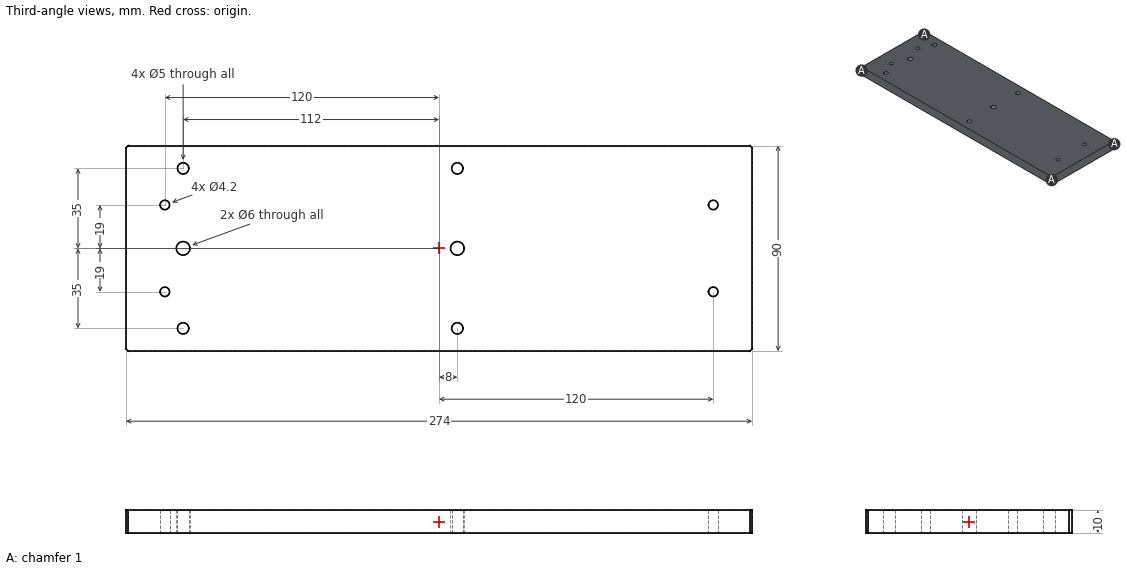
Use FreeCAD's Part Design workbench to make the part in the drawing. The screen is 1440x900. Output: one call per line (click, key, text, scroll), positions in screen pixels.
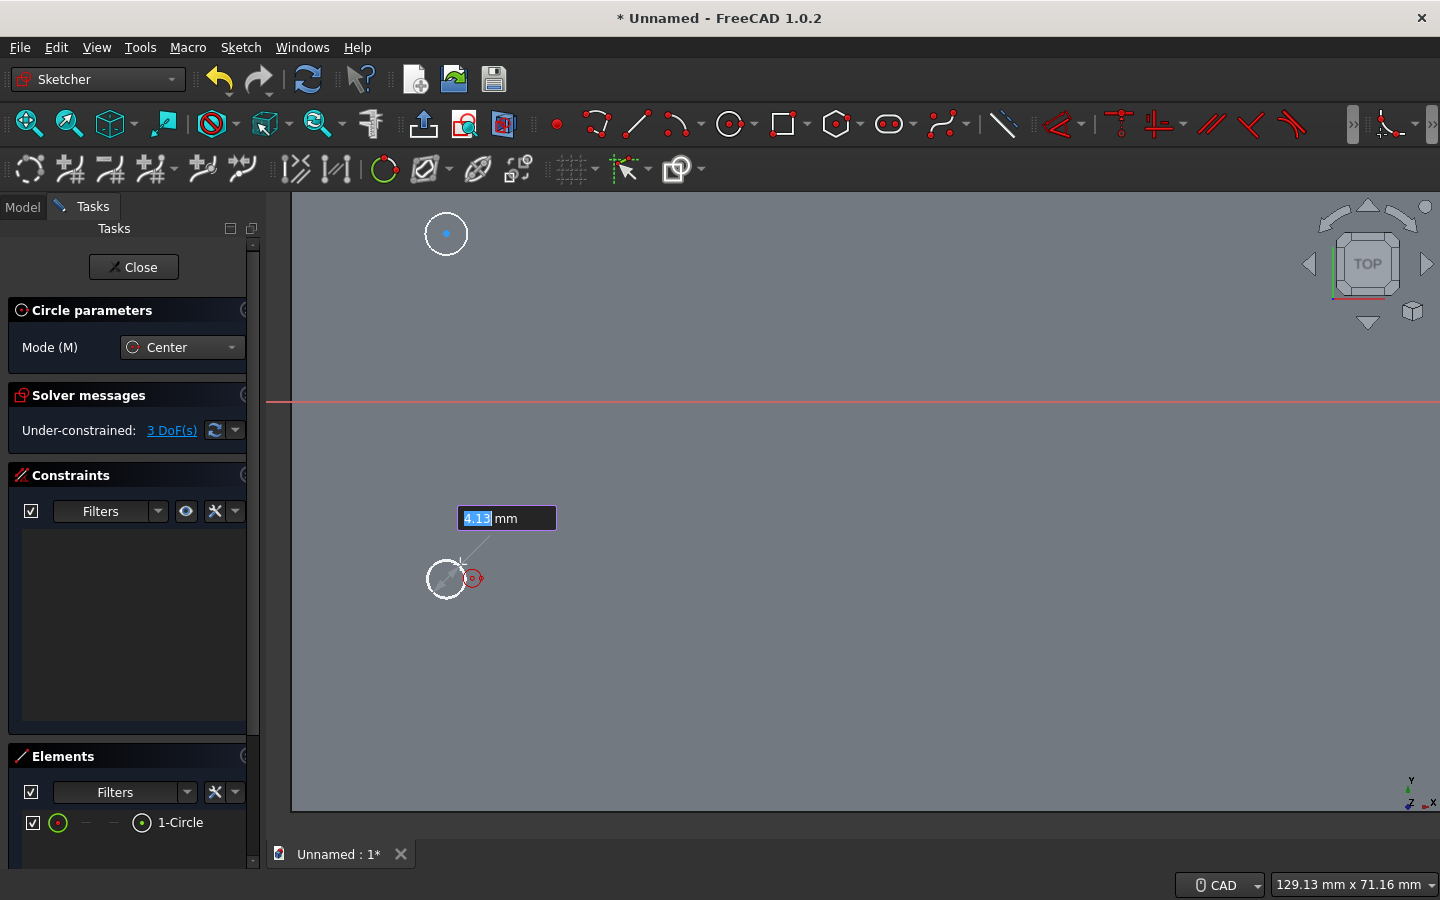
click(459, 562)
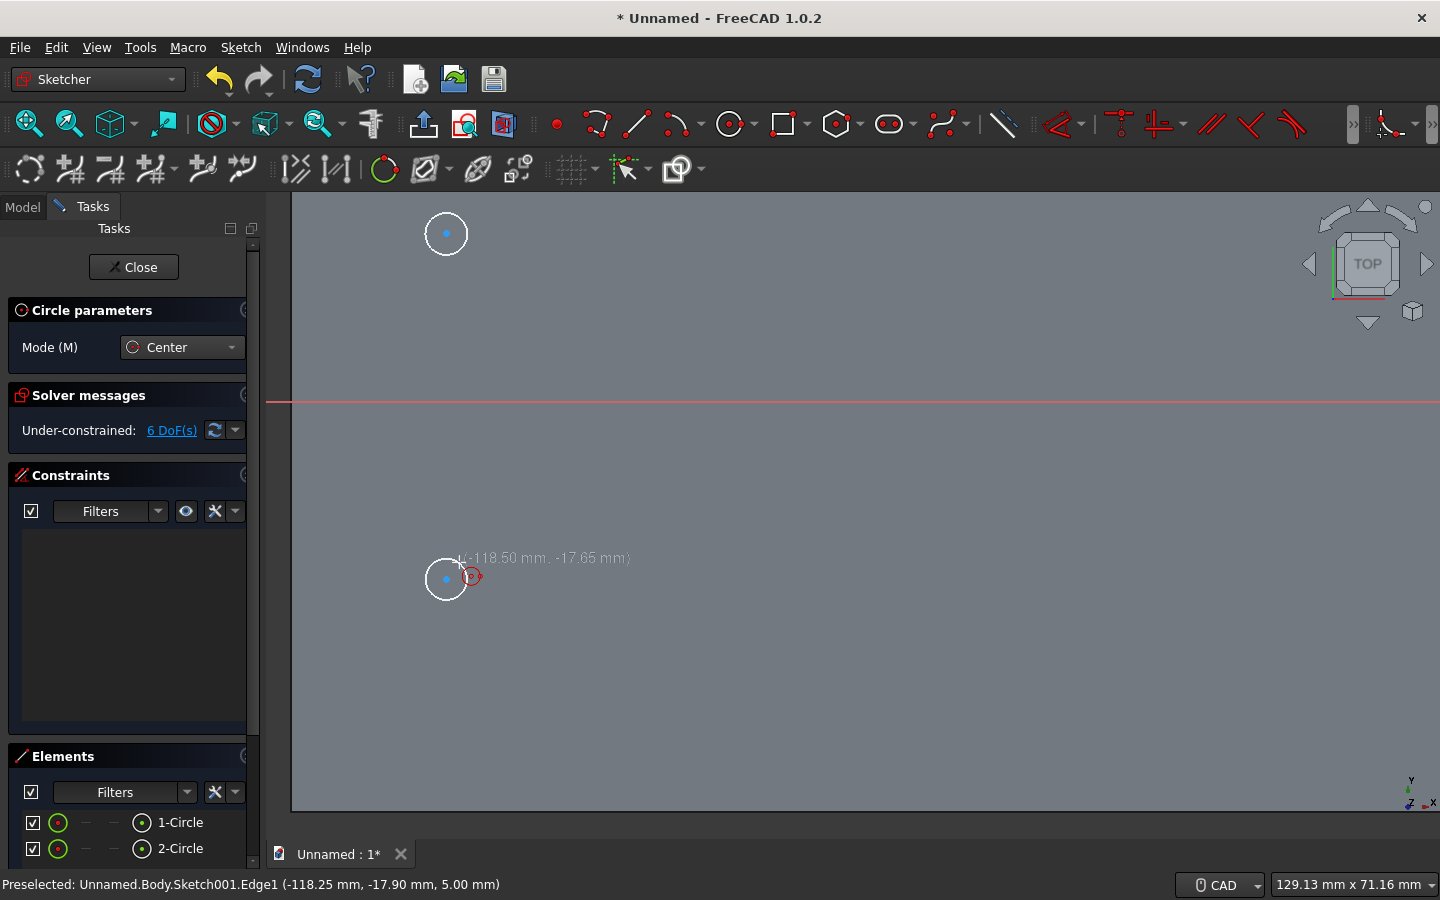
scroll(460, 564, down, 6)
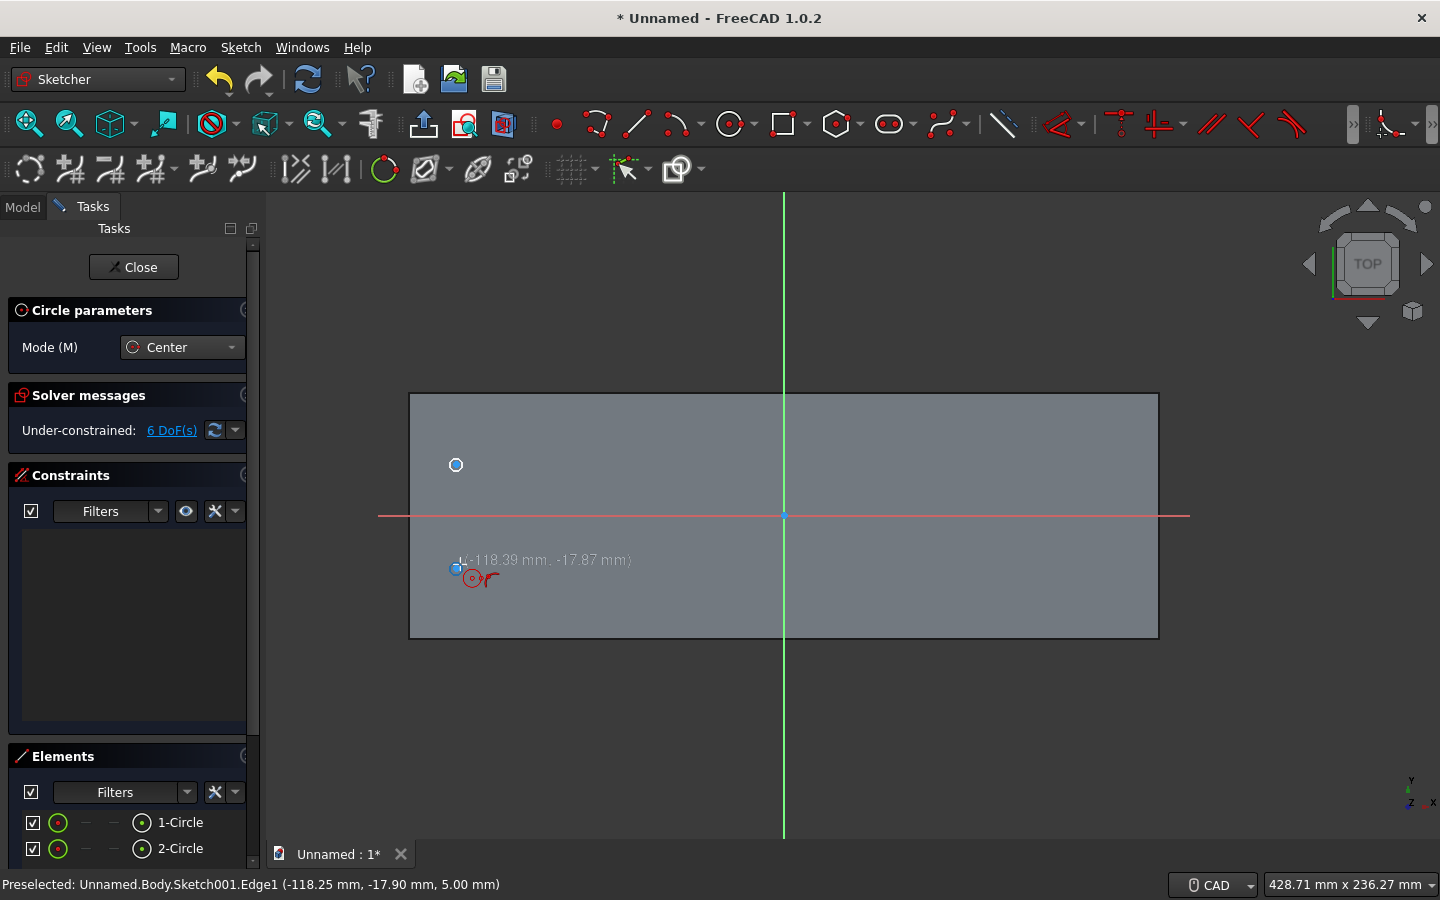
scroll(1113, 568, up, 7)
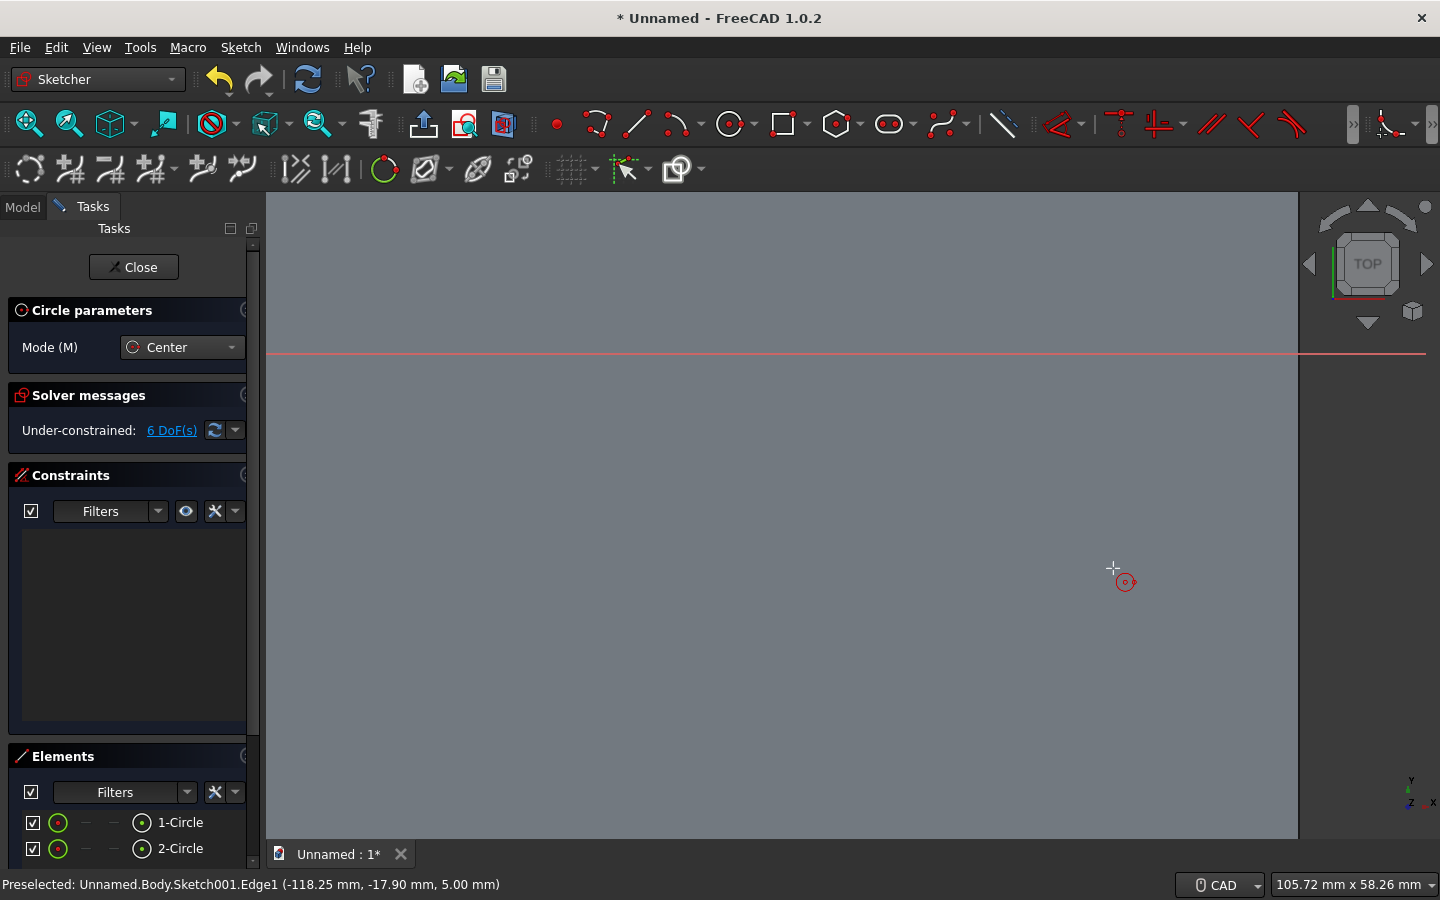
scroll(1114, 568, down, 7)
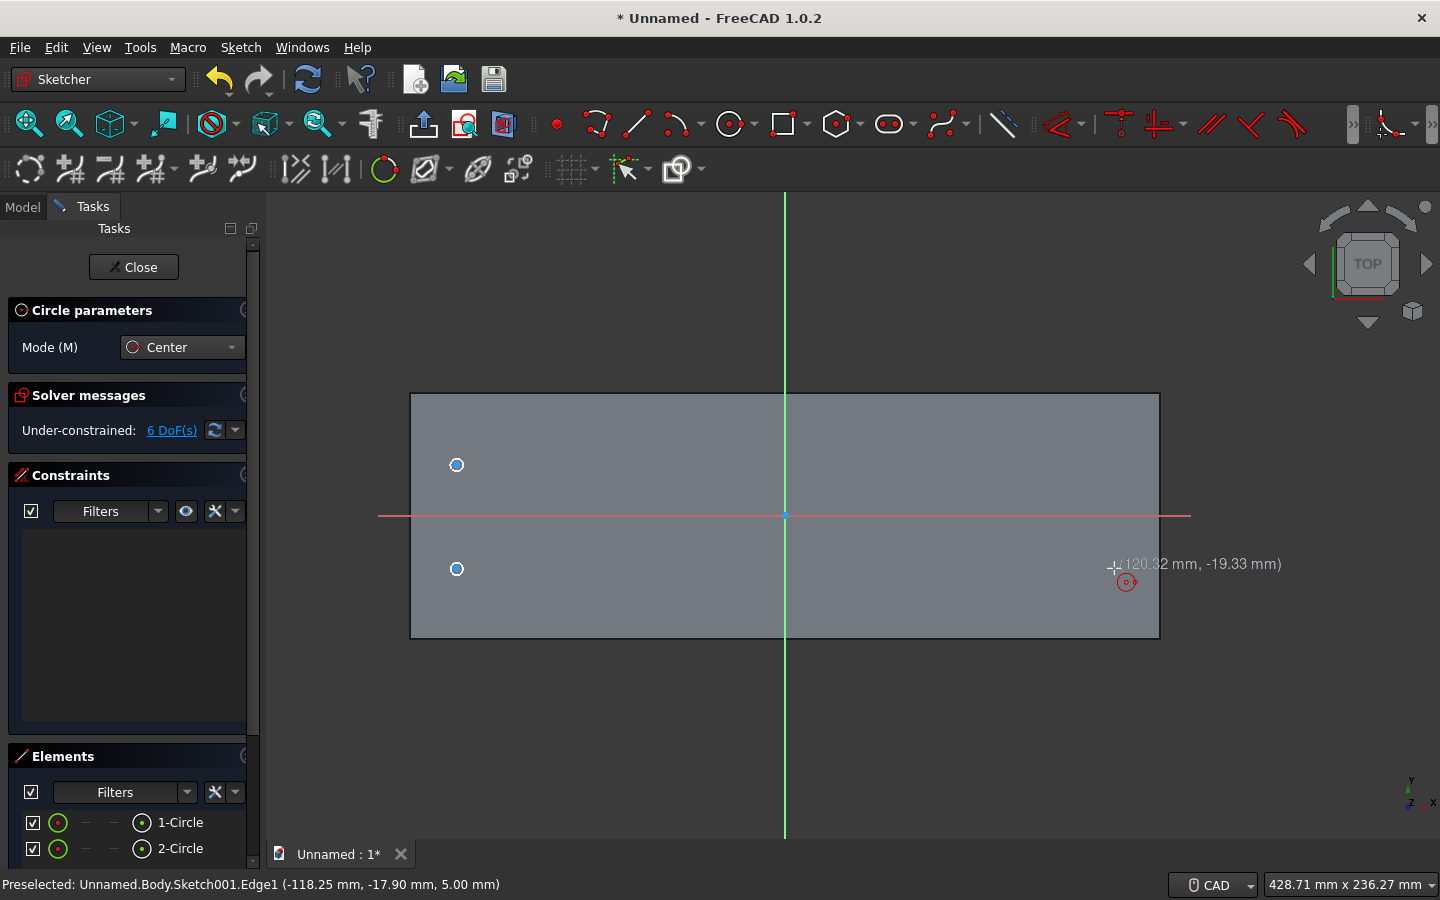
click(1114, 568)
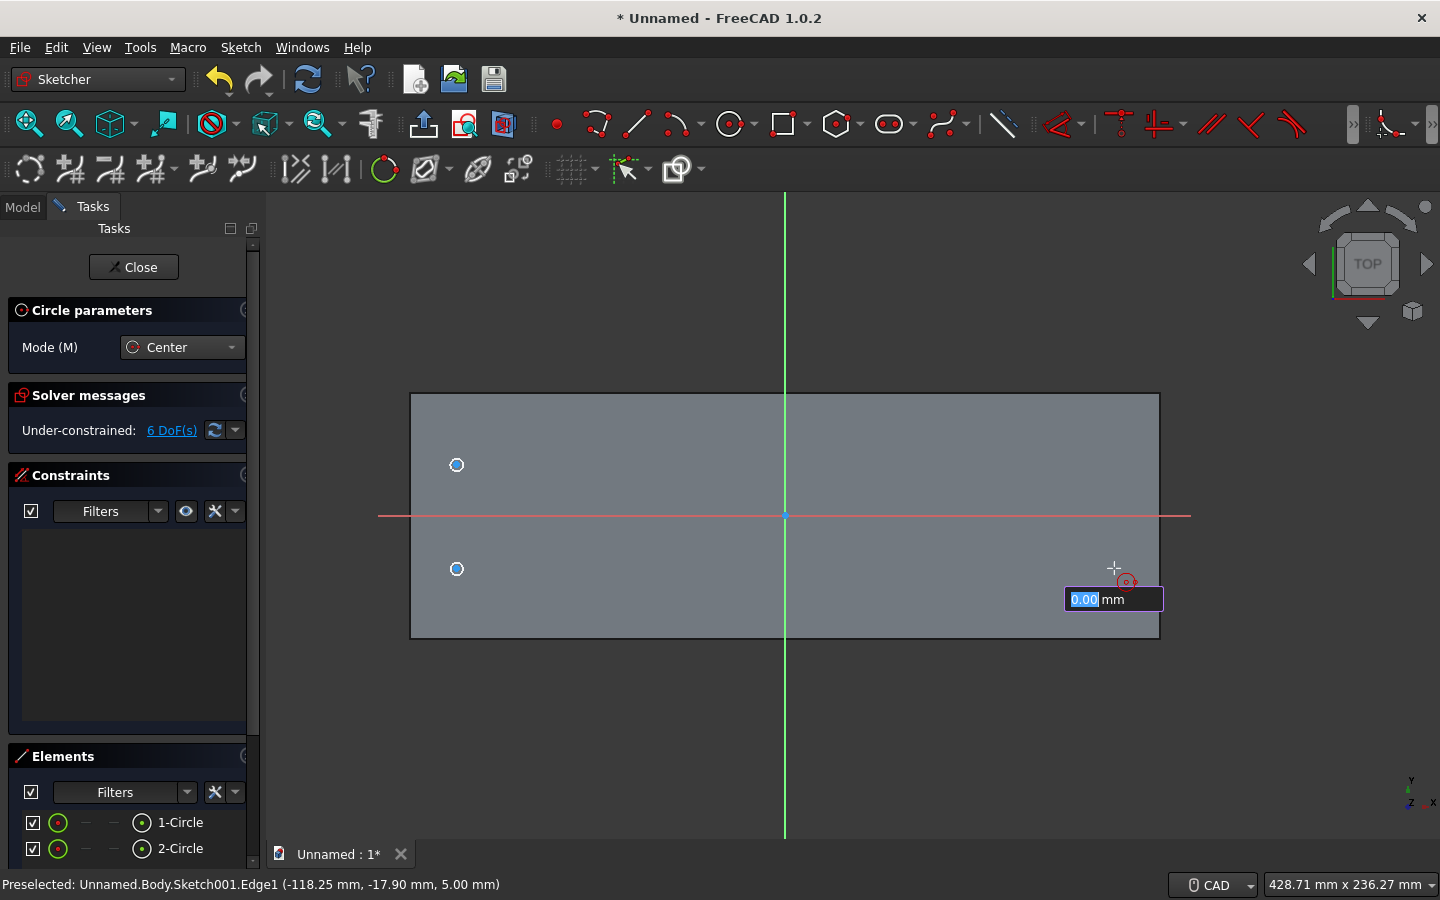
scroll(1118, 564, up, 6)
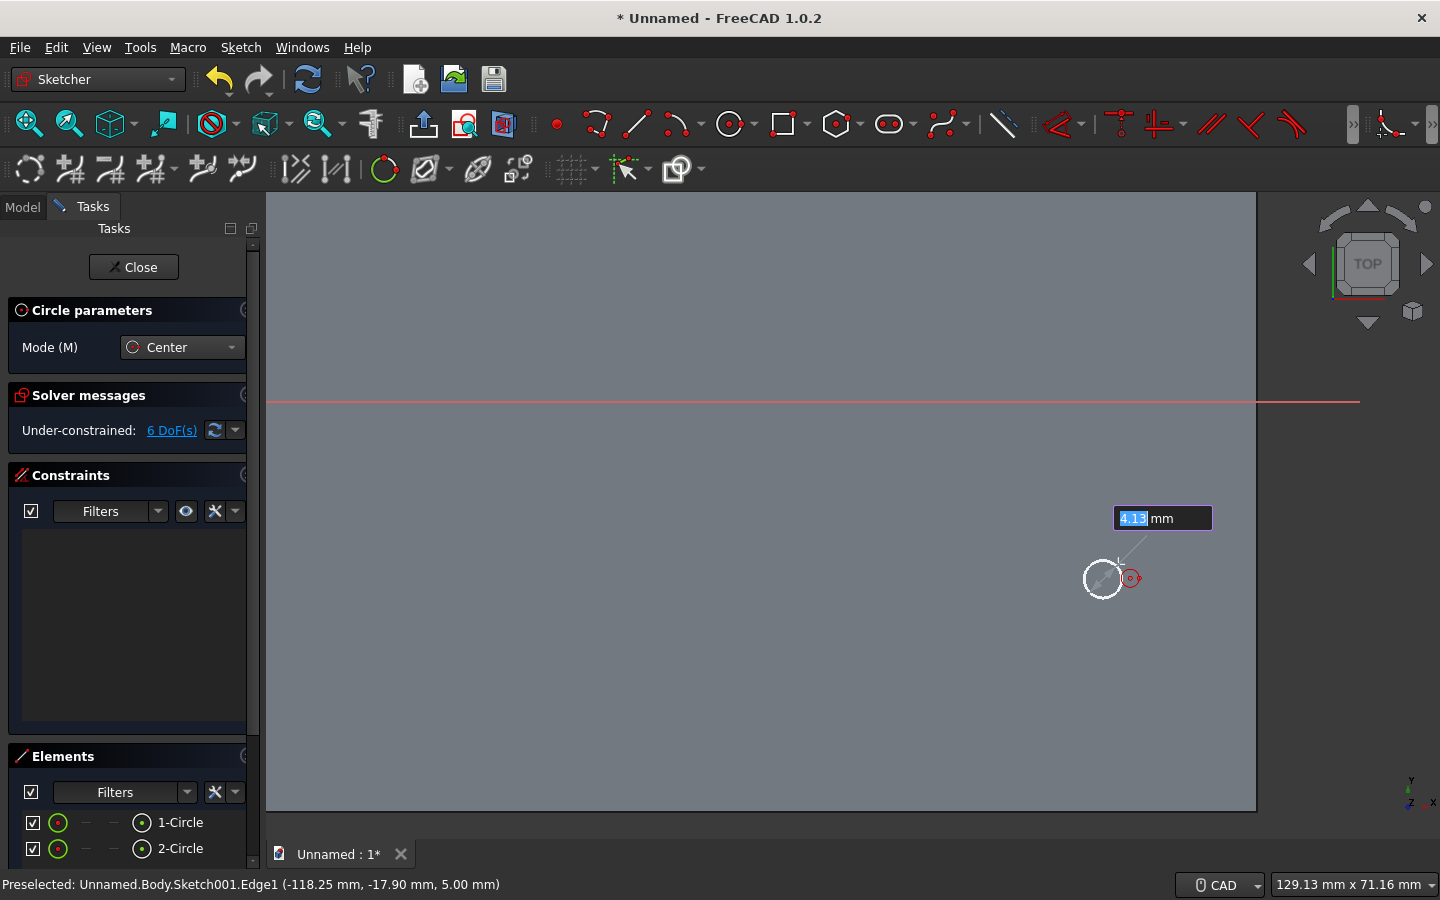
click(1115, 562)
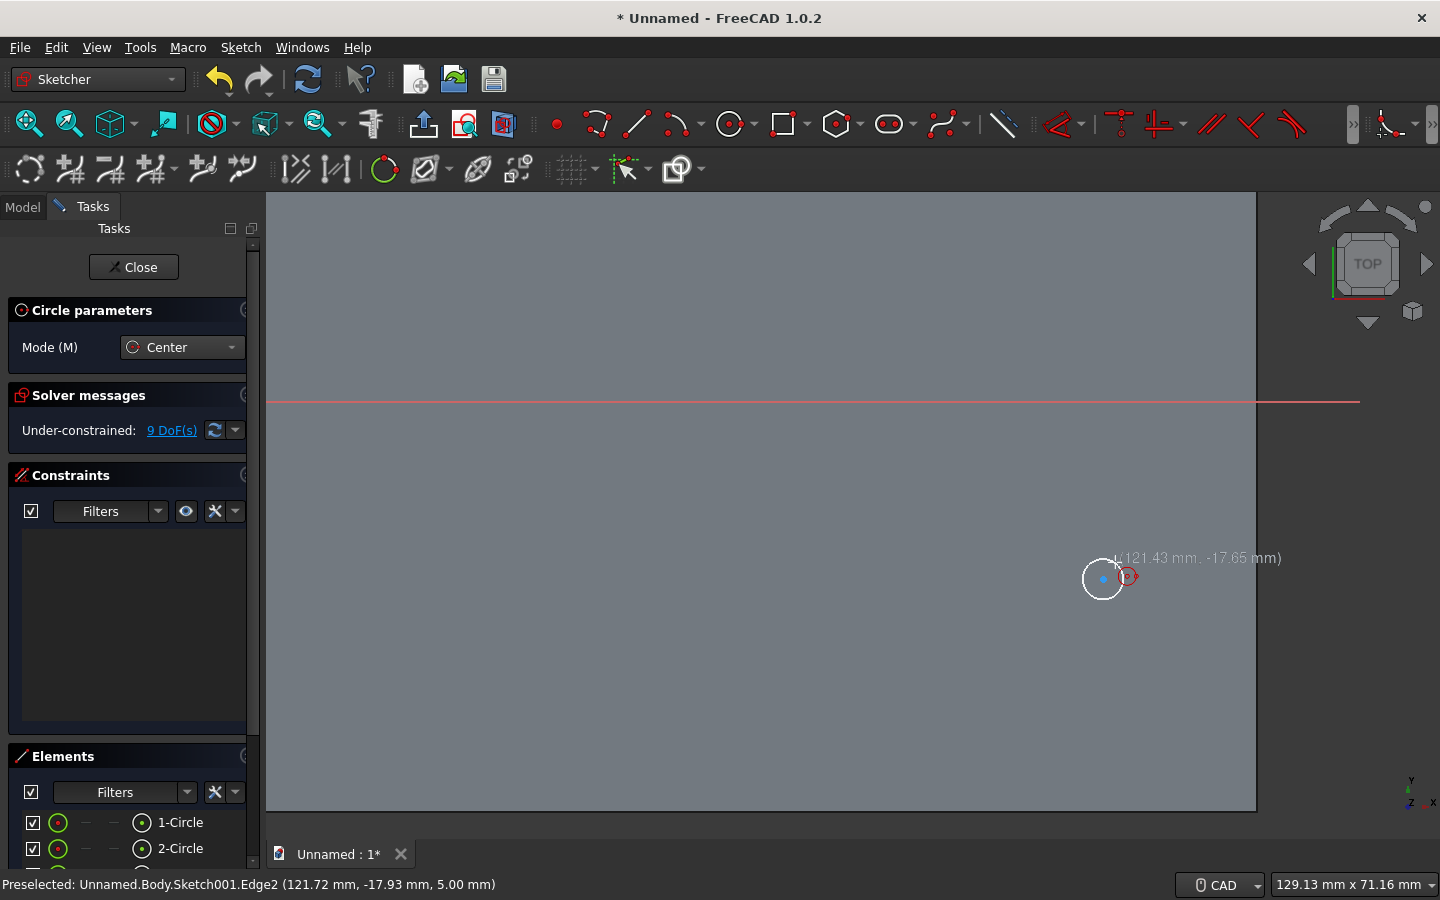
scroll(1118, 564, down, 6)